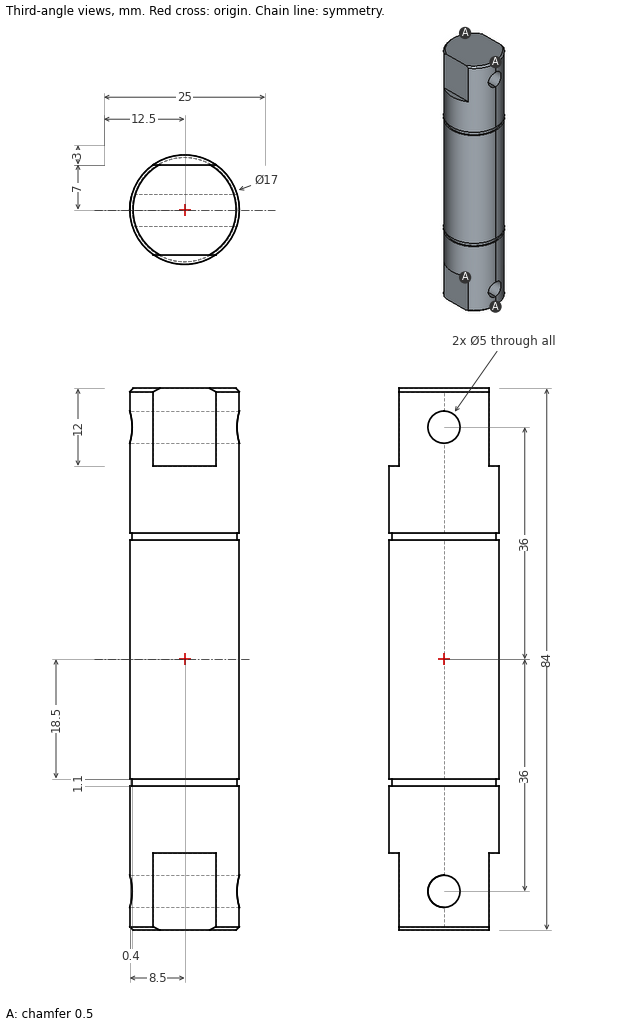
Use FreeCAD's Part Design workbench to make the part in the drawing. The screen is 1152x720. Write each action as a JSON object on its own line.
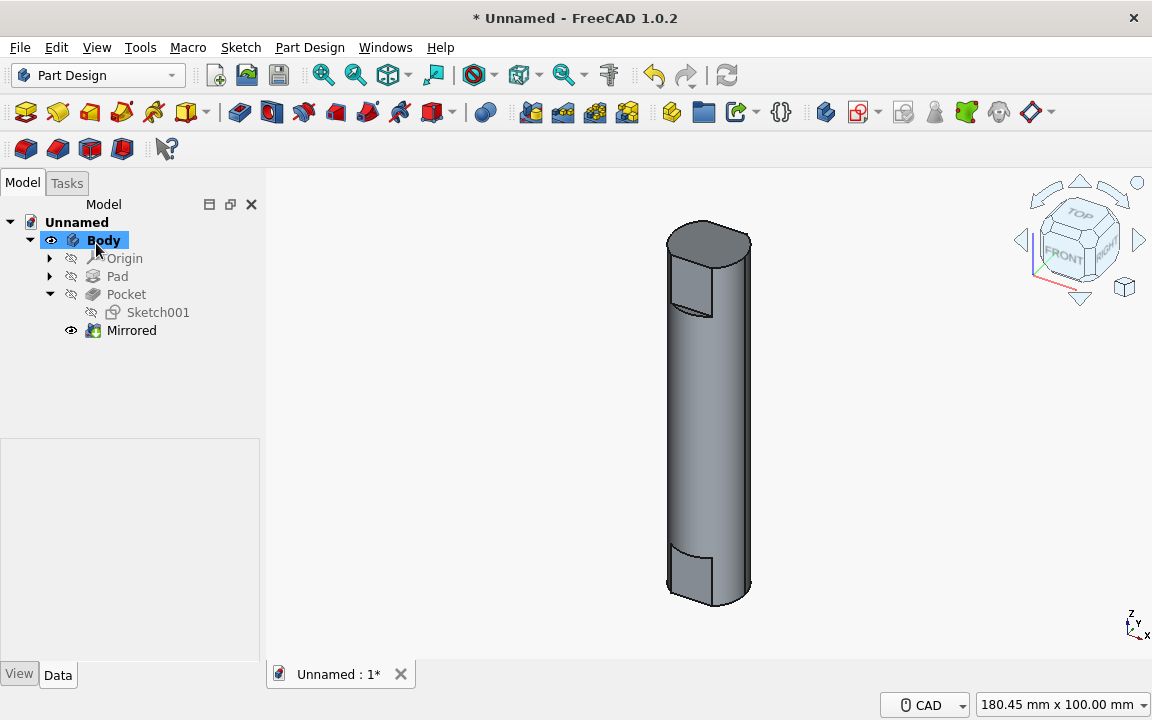
{"action": "left_click", "coordinate": [731, 264]}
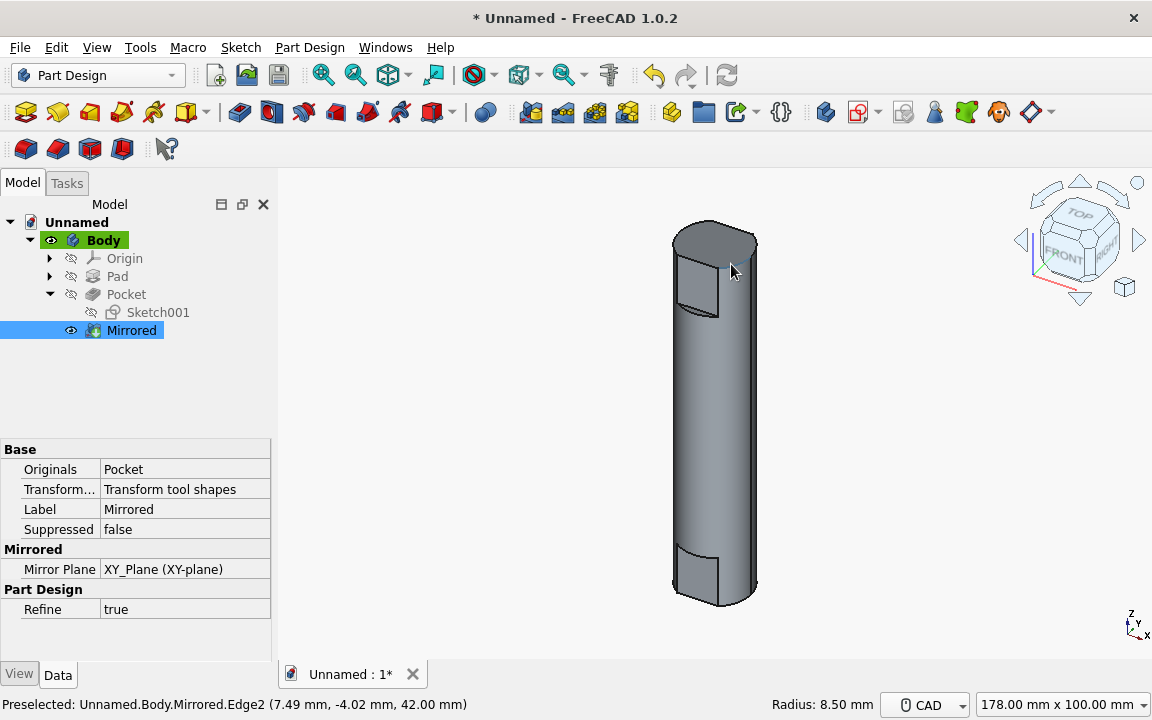
{"action": "left_click", "coordinate": [674, 240], "text": "ctrl"}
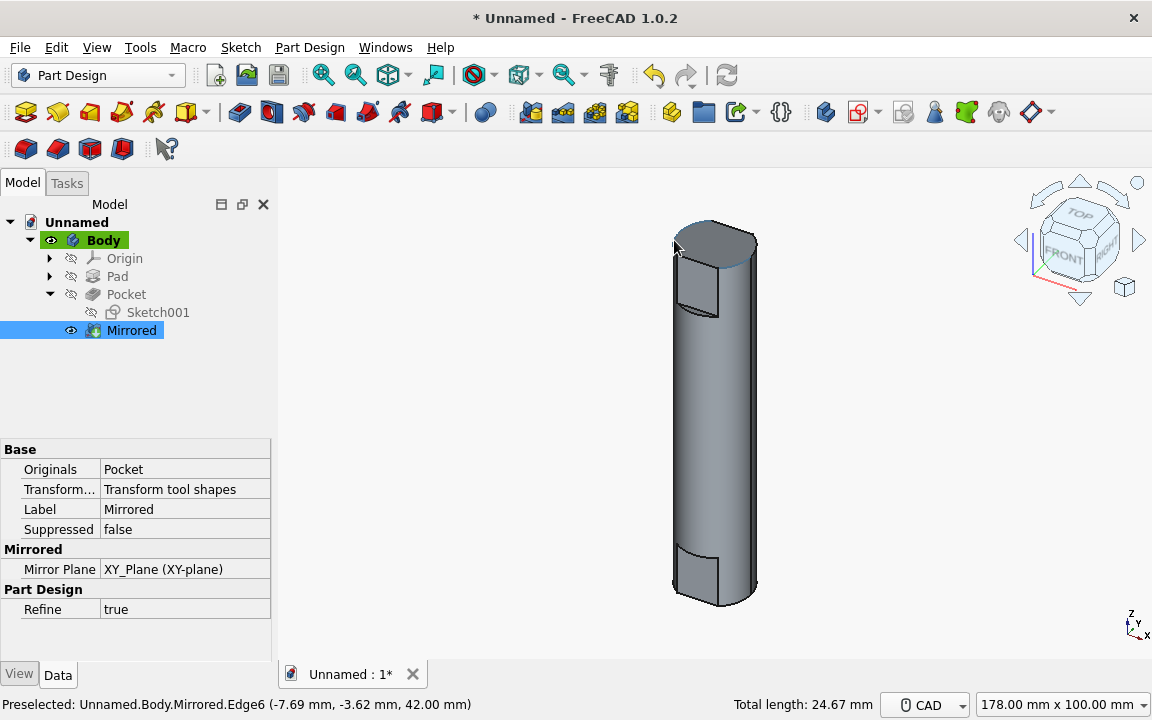
{"action": "key", "text": "0"}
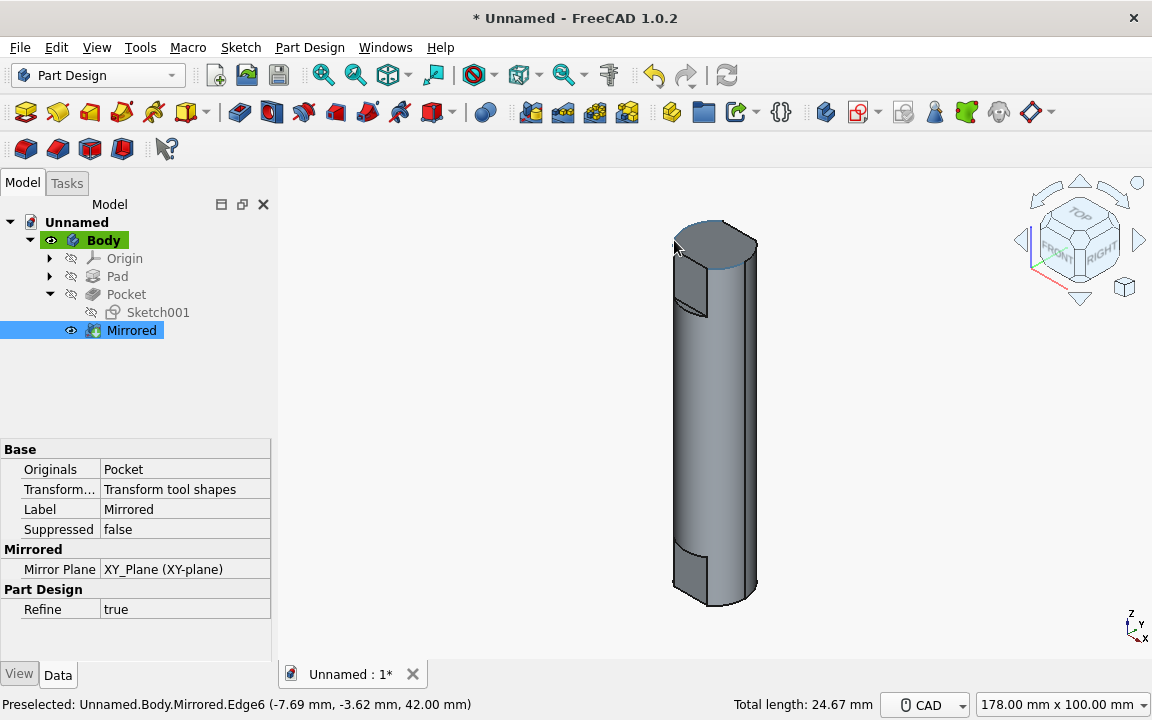
{"action": "key", "text": "2"}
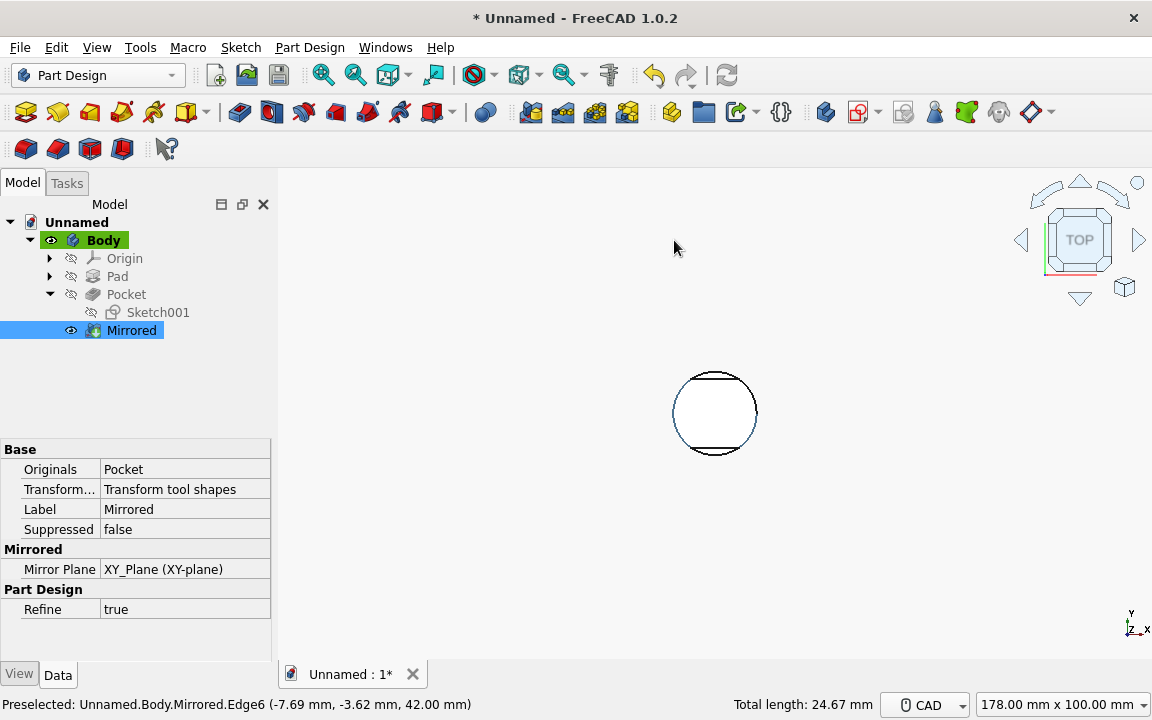
{"action": "left_click", "coordinate": [324, 76]}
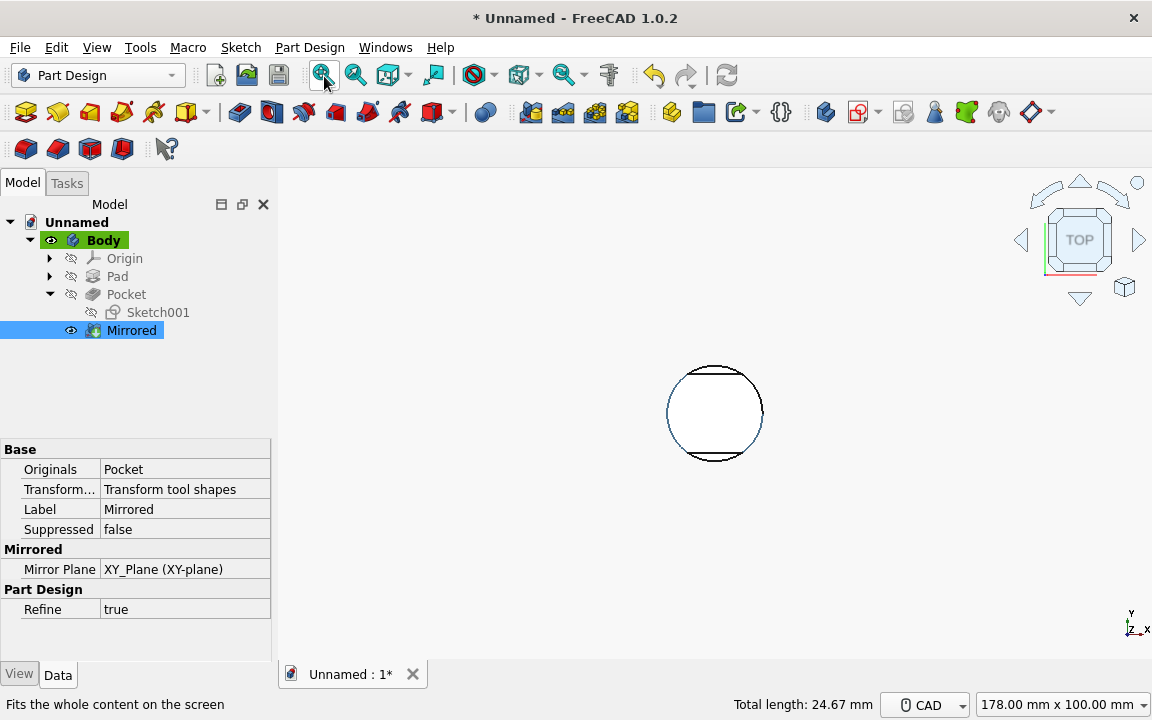
{"action": "key", "text": "1"}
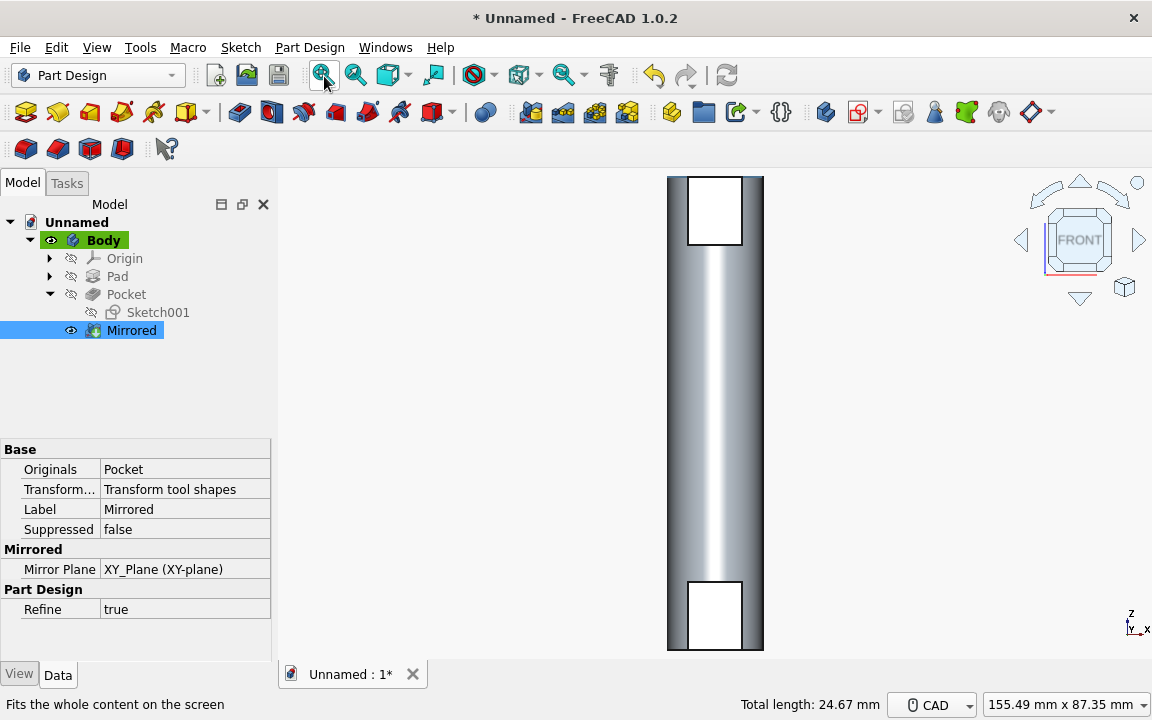
{"action": "key", "text": "3"}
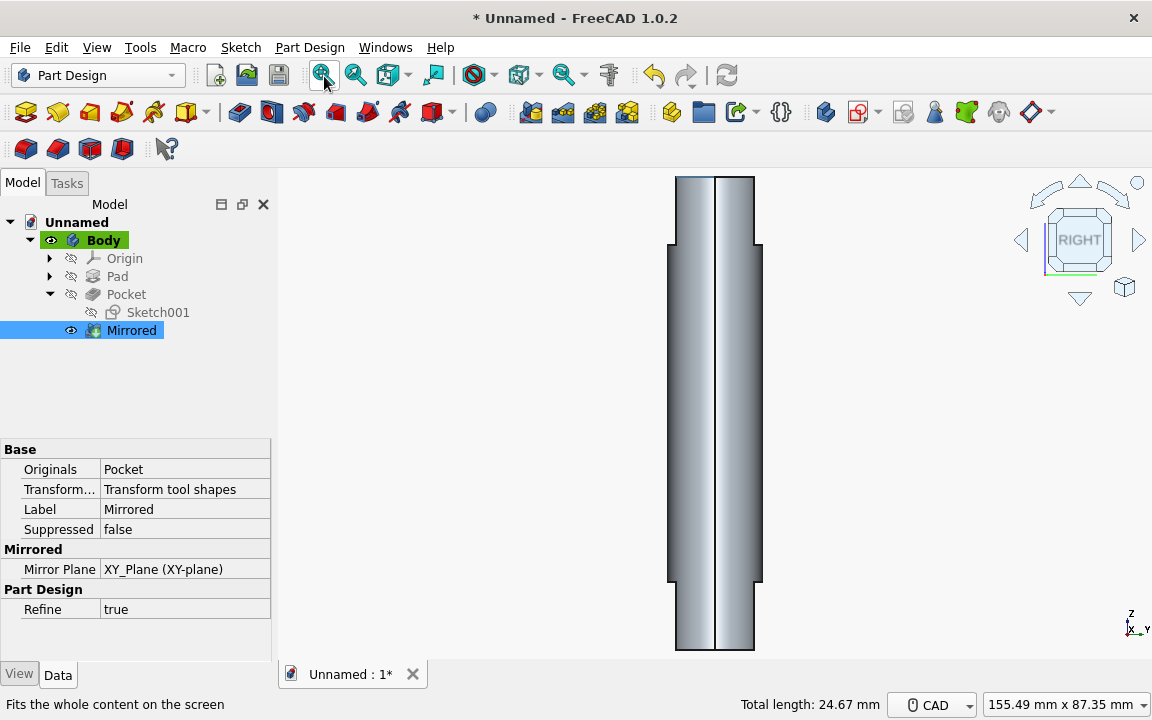
{"action": "key", "text": "5"}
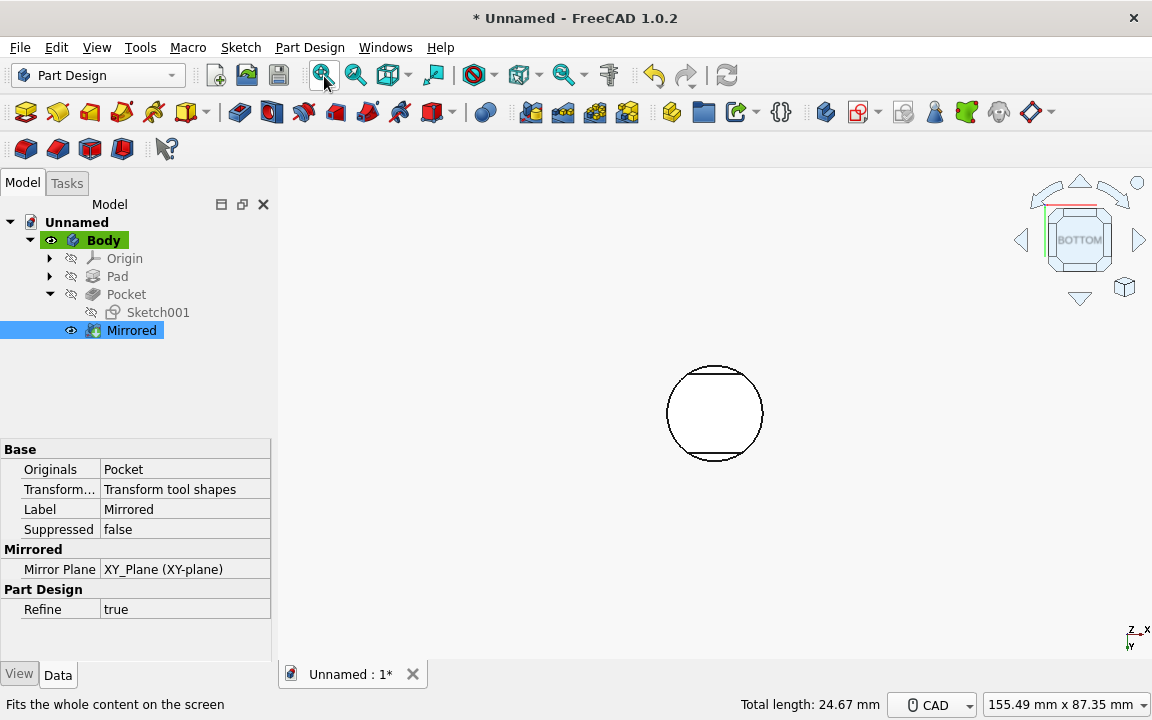
{"action": "left_click", "coordinate": [324, 76]}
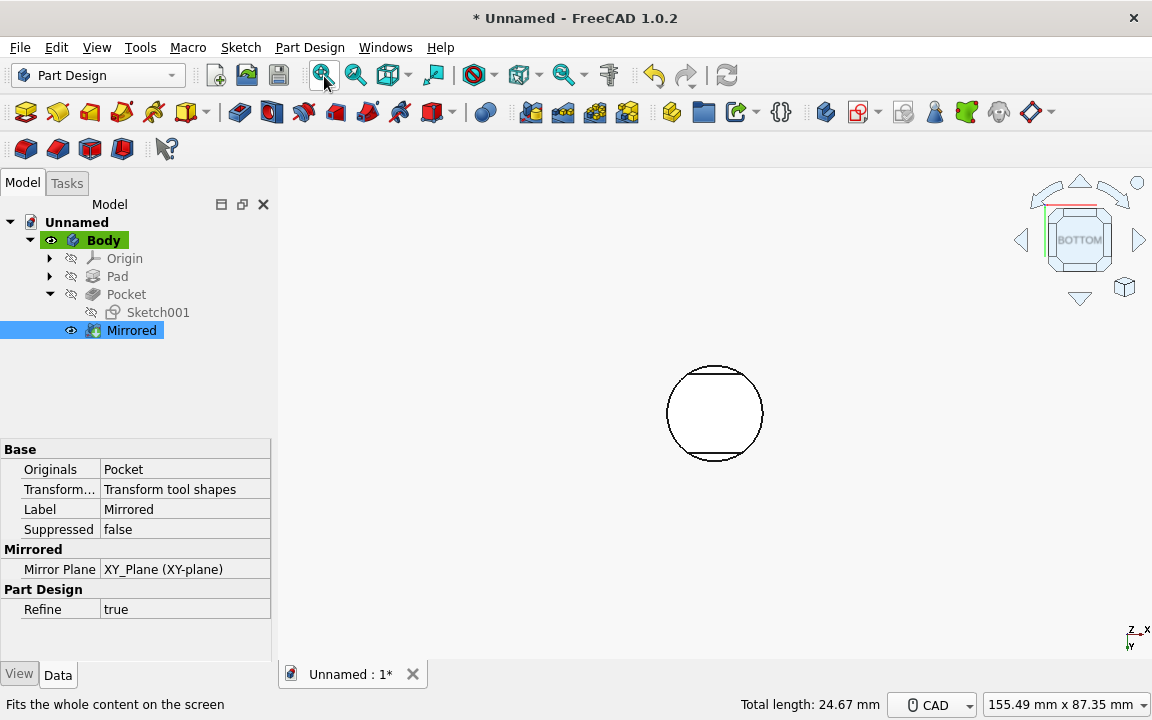
{"action": "left_click", "coordinate": [667, 412], "text": "ctrl"}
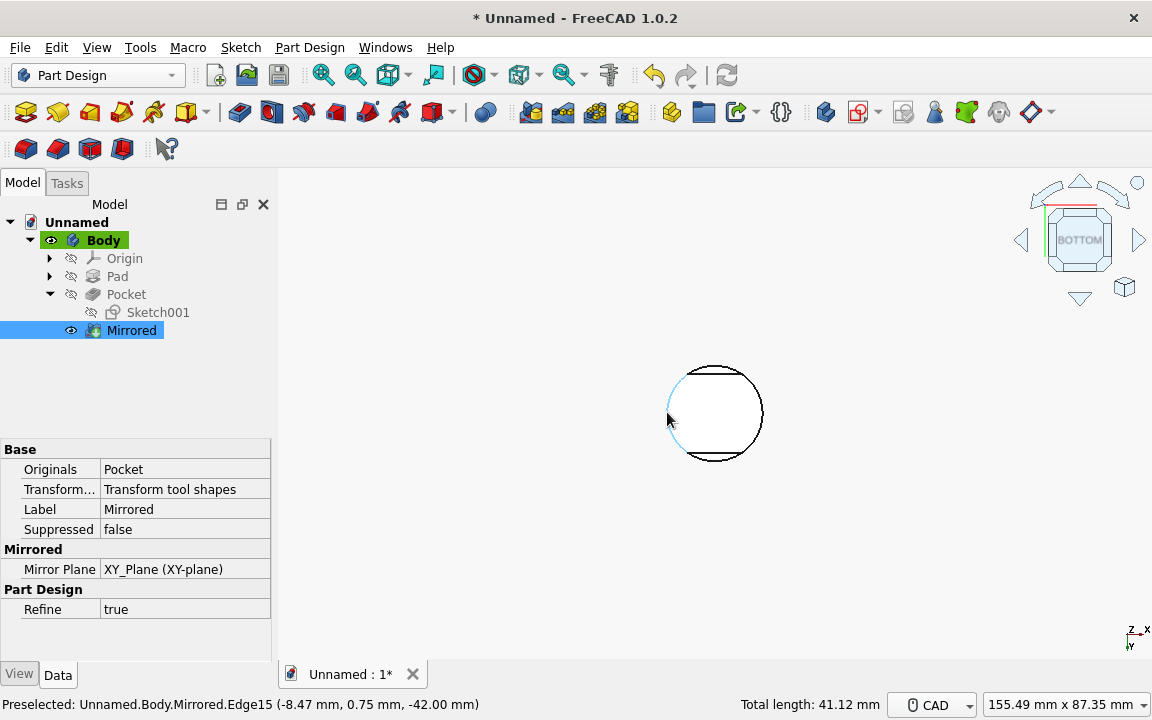
{"action": "left_click", "coordinate": [757, 435], "text": "ctrl"}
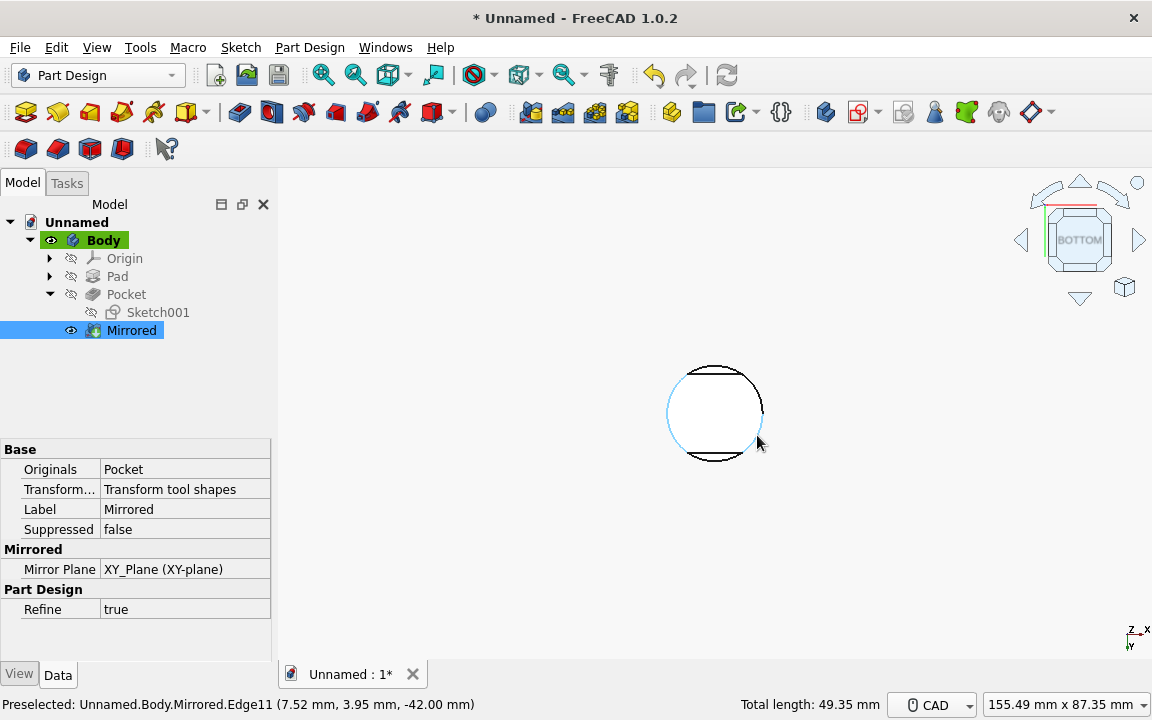
{"action": "left_click", "coordinate": [58, 150]}